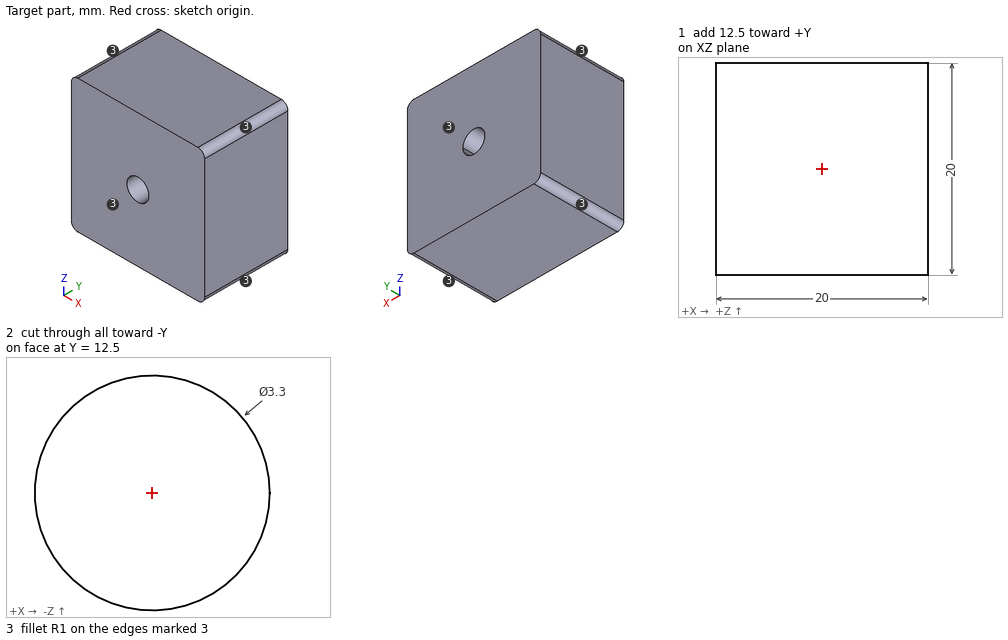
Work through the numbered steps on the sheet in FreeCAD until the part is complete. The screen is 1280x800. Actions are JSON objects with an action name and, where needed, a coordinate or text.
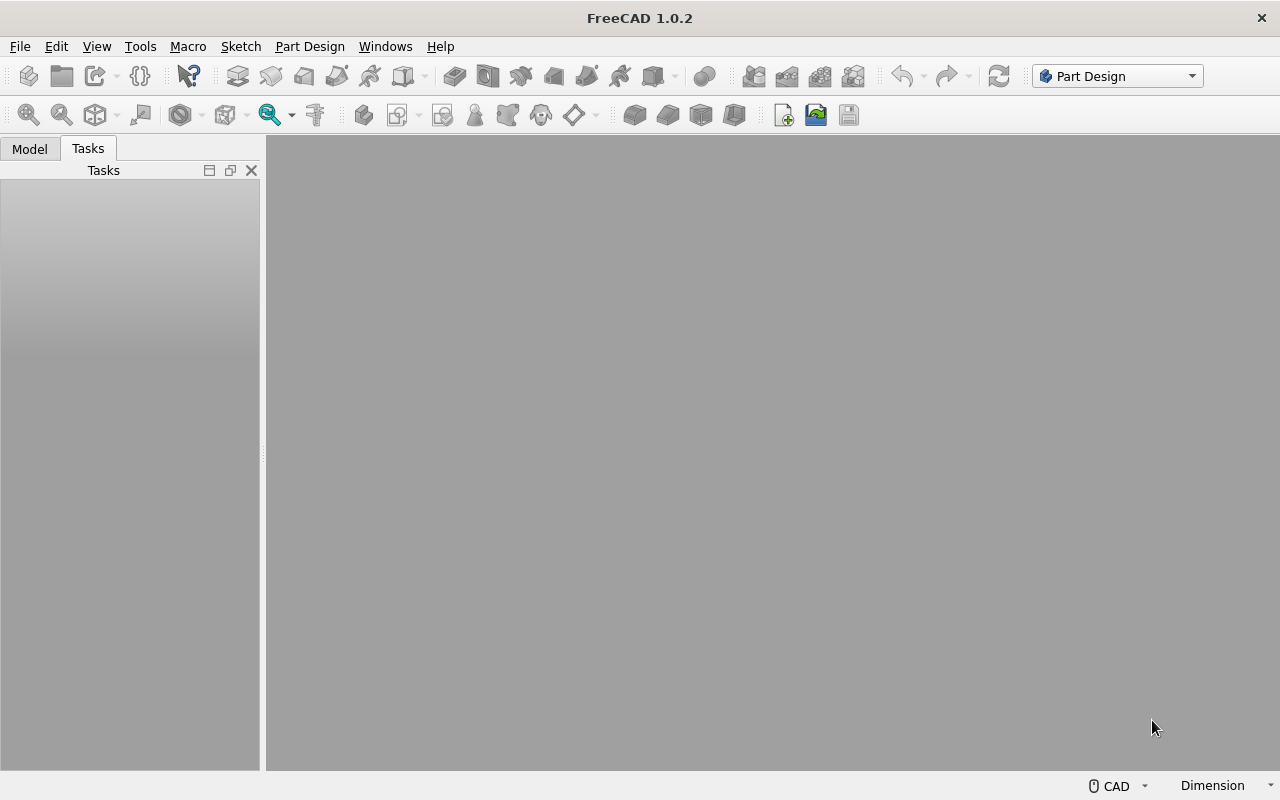
{"action": "left_click", "coordinate": [783, 116]}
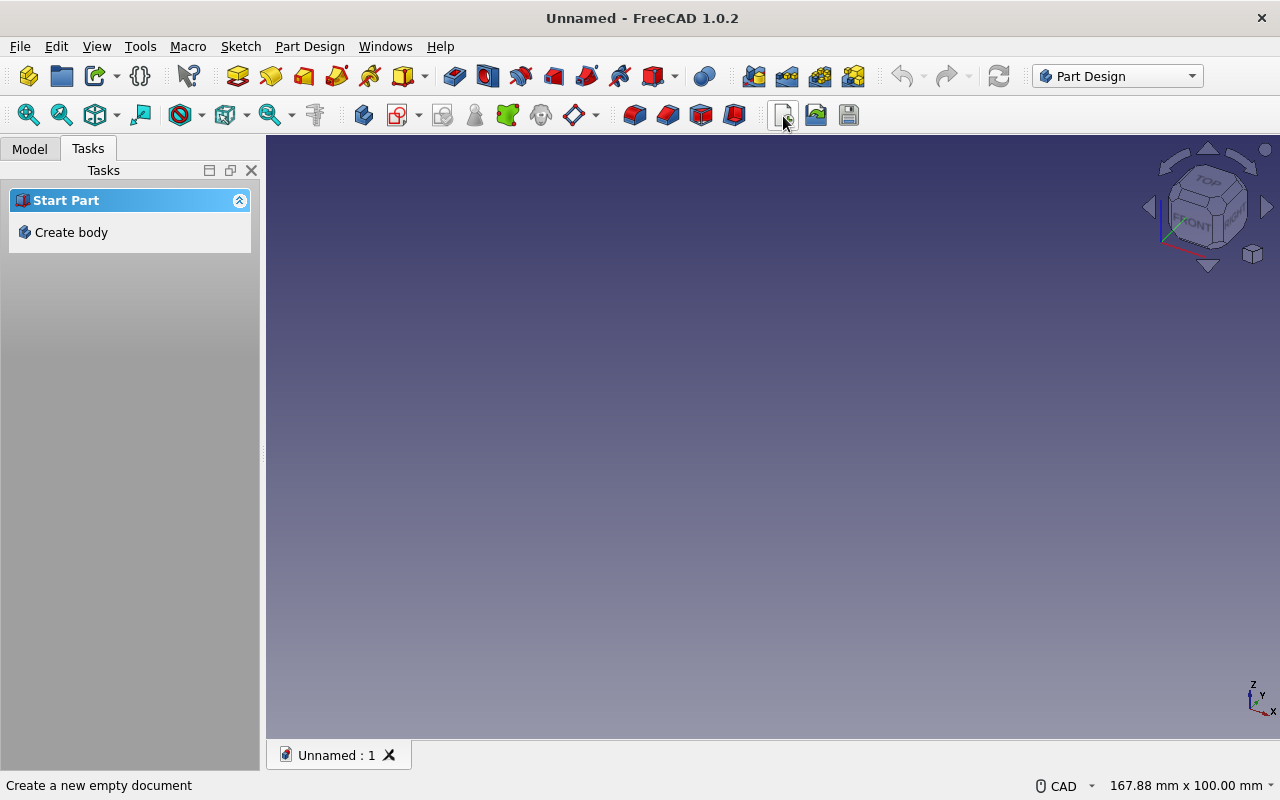
{"action": "left_click", "coordinate": [396, 116]}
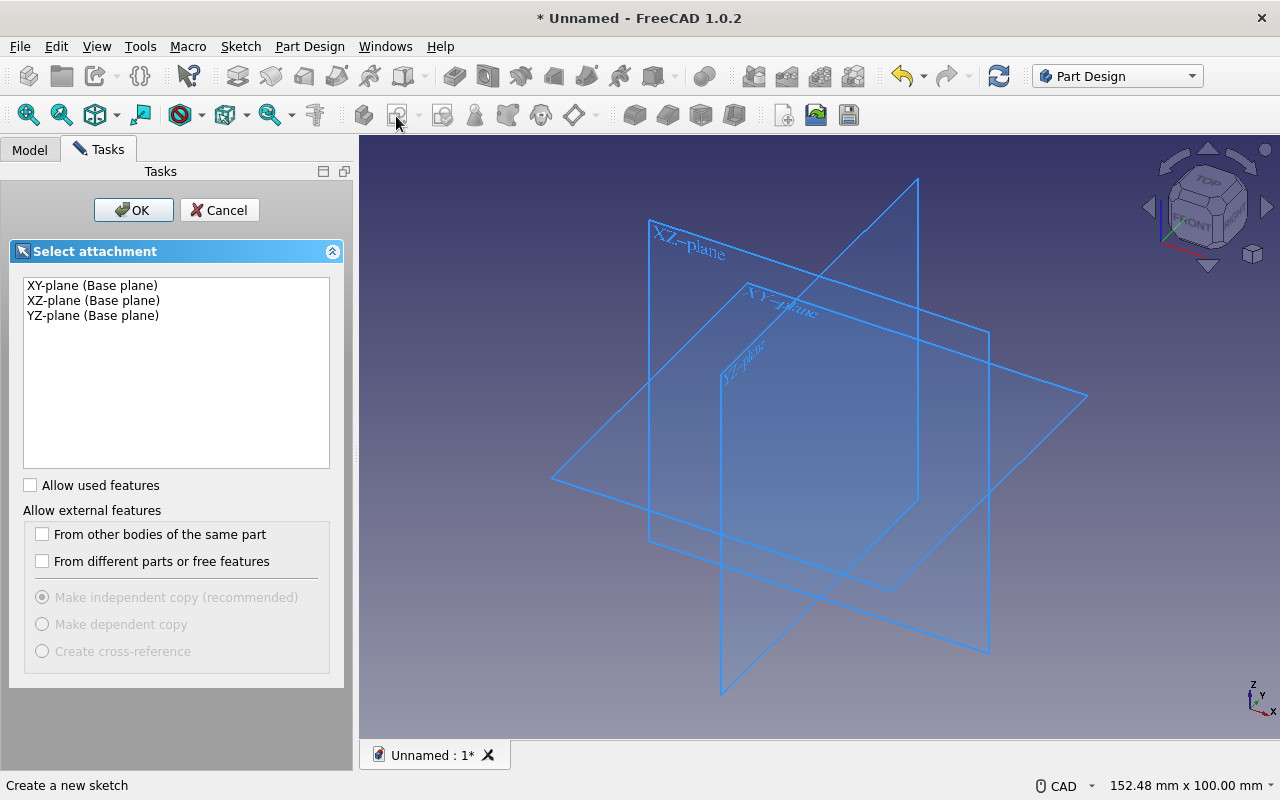
{"action": "left_click", "coordinate": [84, 300]}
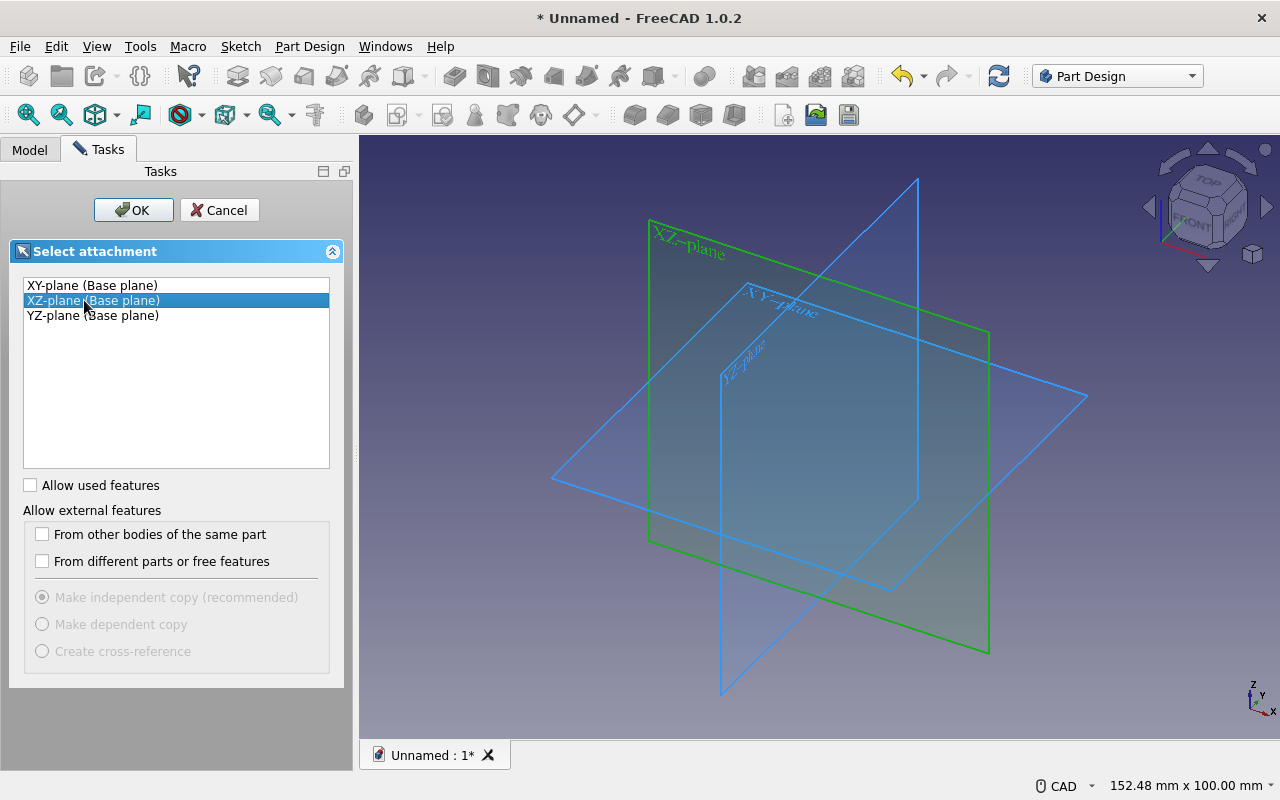
{"action": "left_click", "coordinate": [134, 210]}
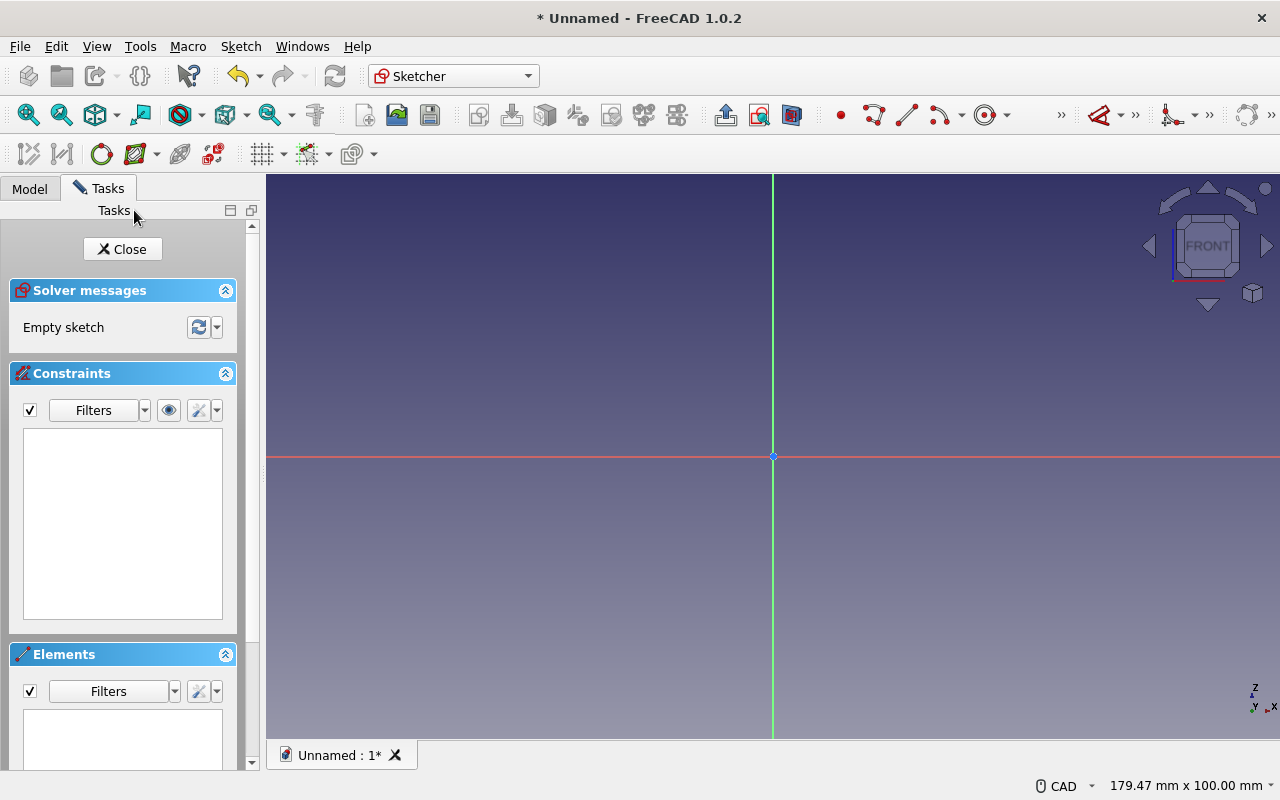
{"action": "scroll", "coordinate": [803, 456], "scroll_direction": "up", "scroll_amount": 6}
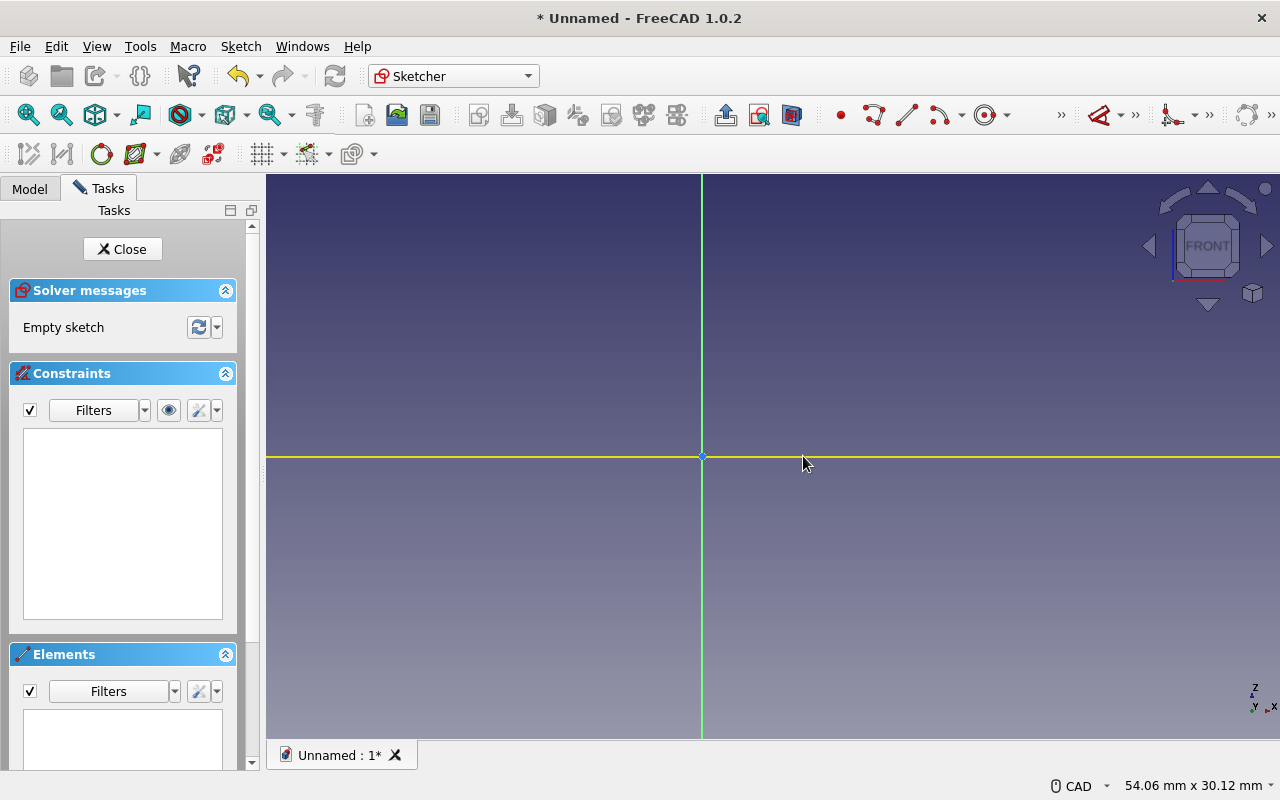
{"action": "key", "text": "g v"}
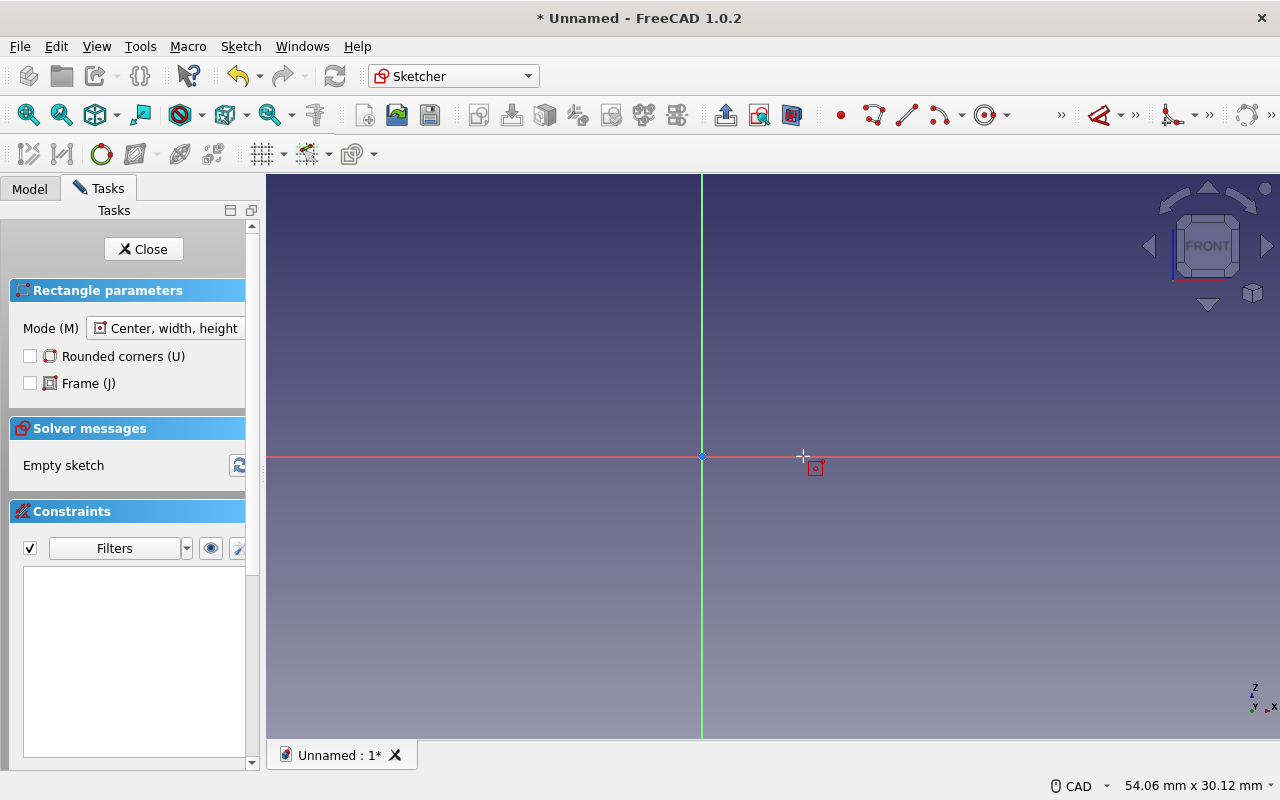
{"action": "left_click", "coordinate": [702, 456]}
{"action": "left_click", "coordinate": [890, 269]}
{"action": "key", "text": "Escape"}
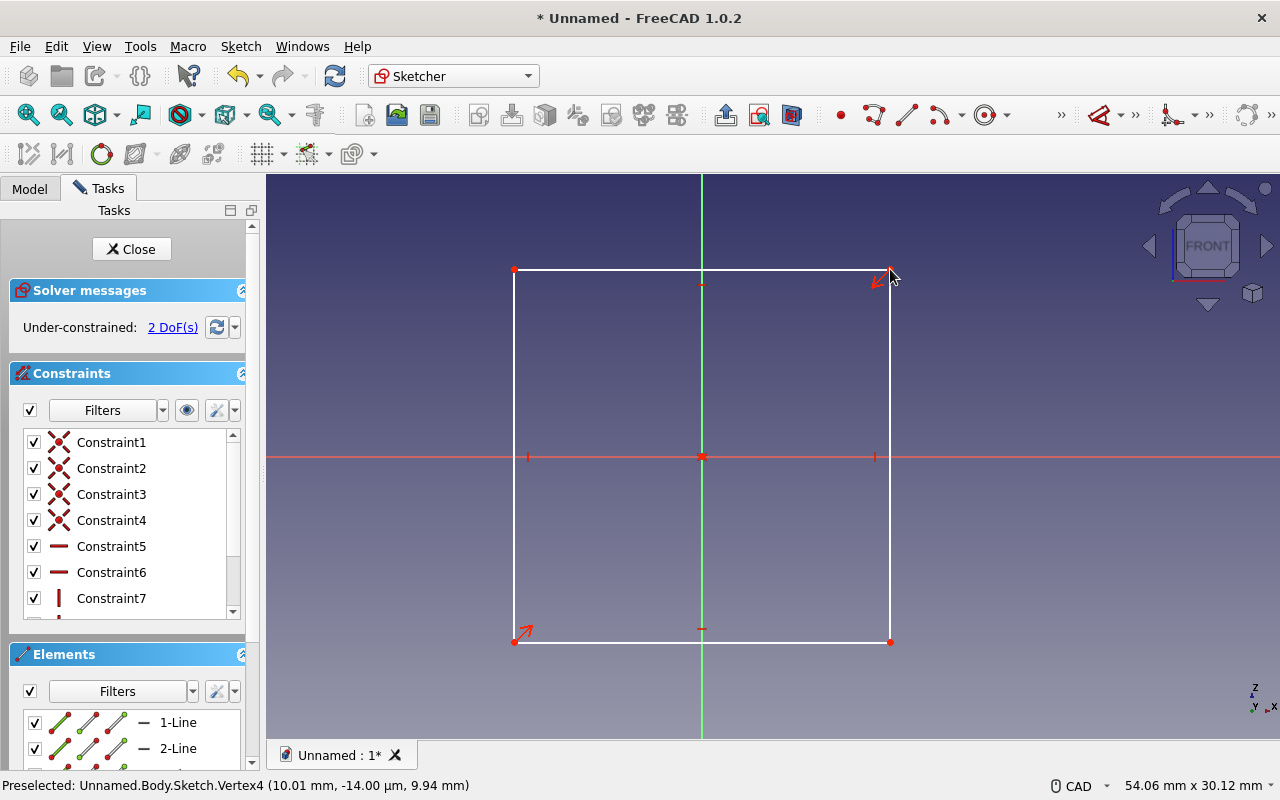
{"action": "left_click", "coordinate": [1098, 116]}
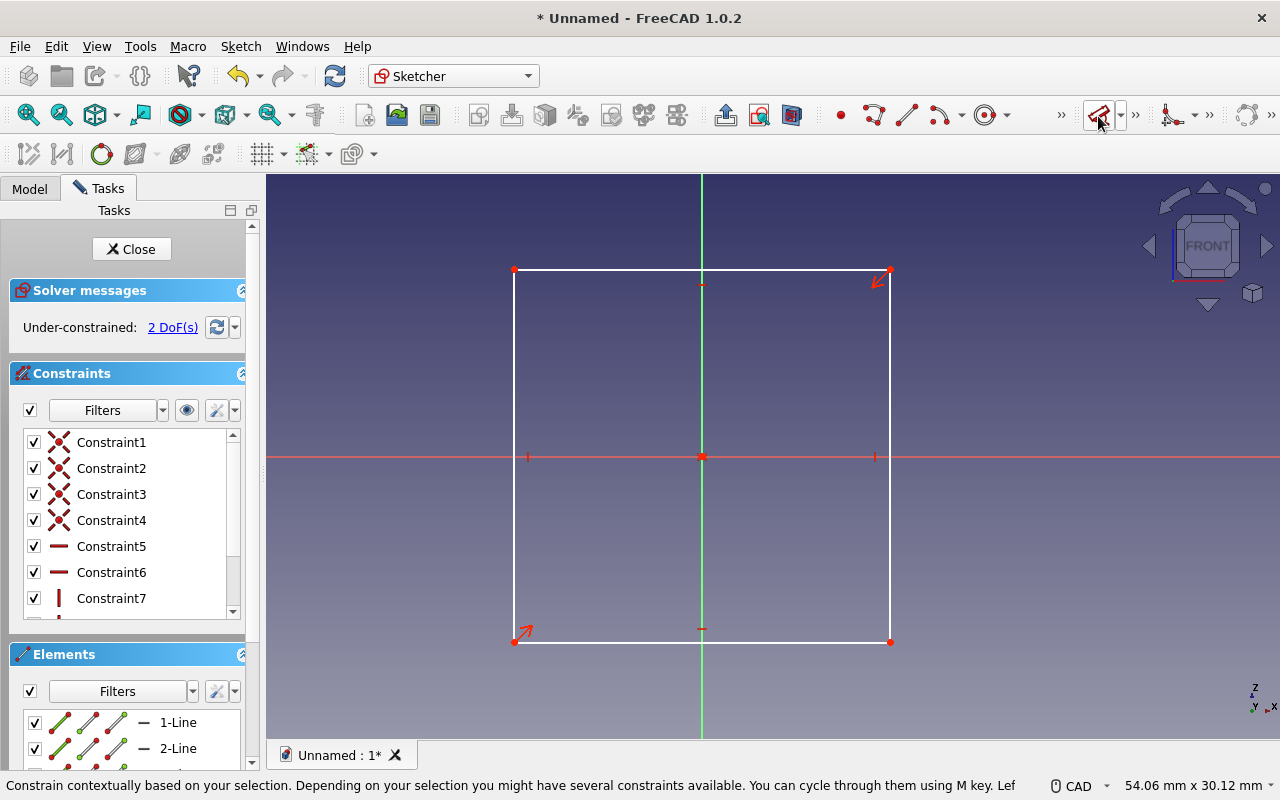
{"action": "left_click", "coordinate": [627, 643]}
{"action": "left_click", "coordinate": [616, 677]}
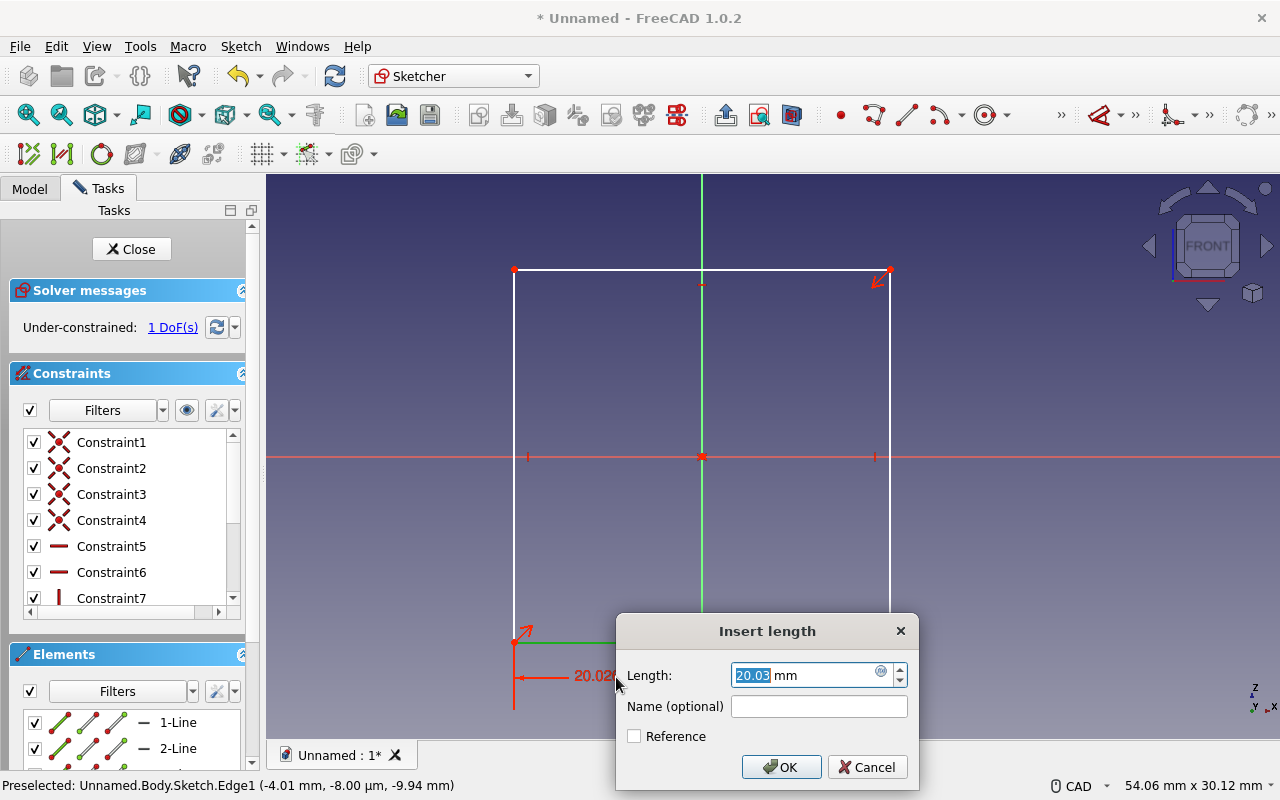
{"action": "type", "text": "20"}
{"action": "key", "text": "Return"}